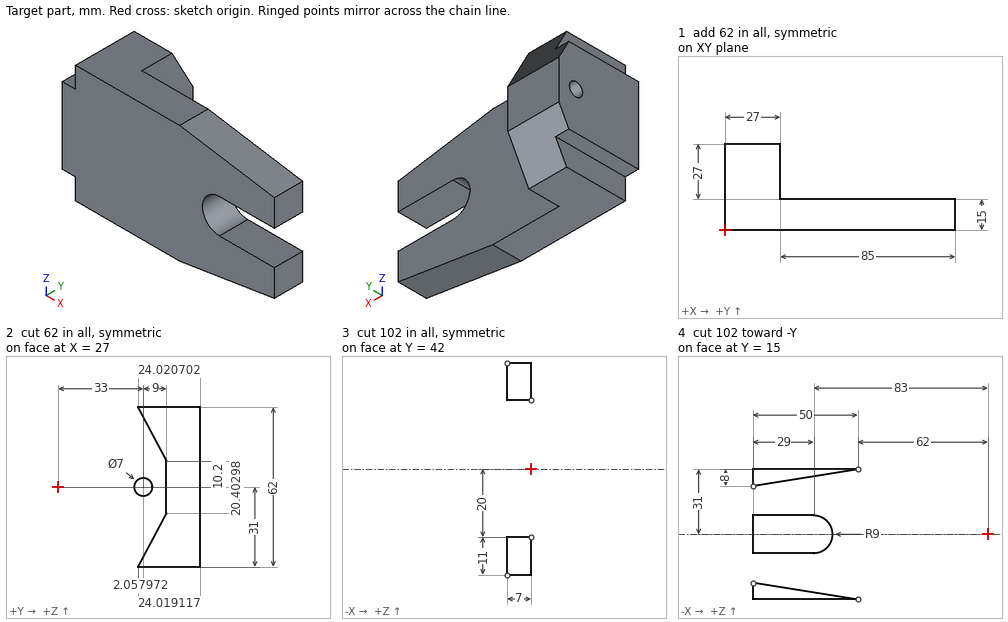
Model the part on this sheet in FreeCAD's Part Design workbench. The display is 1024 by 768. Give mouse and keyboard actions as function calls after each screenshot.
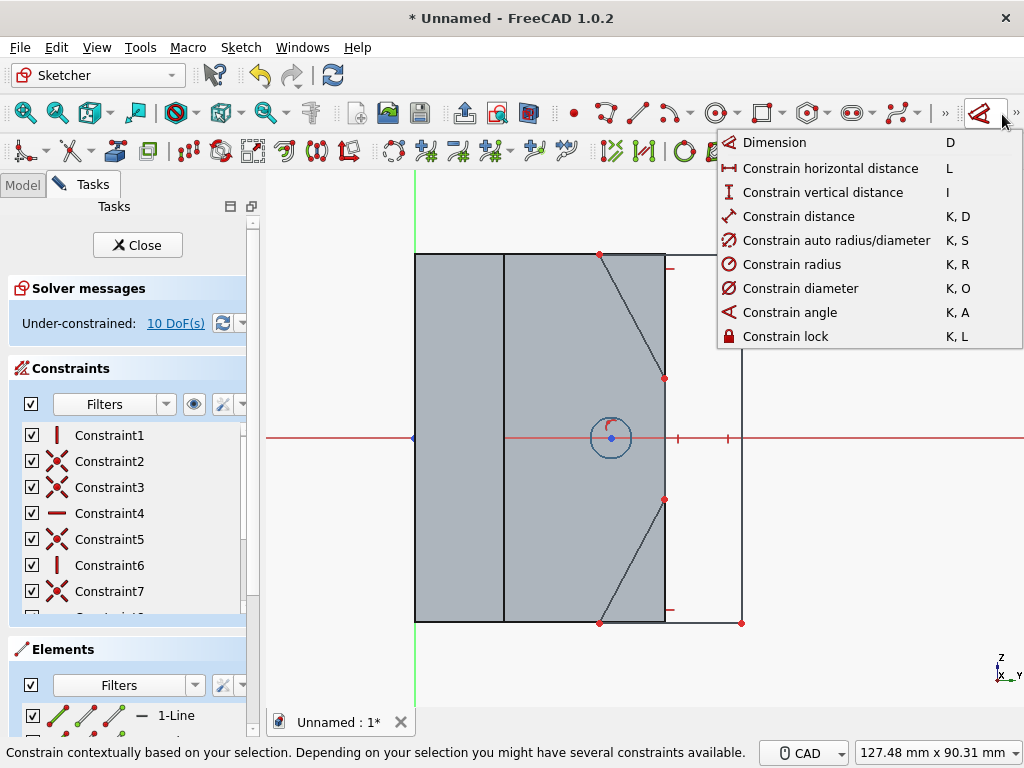
click(870, 288)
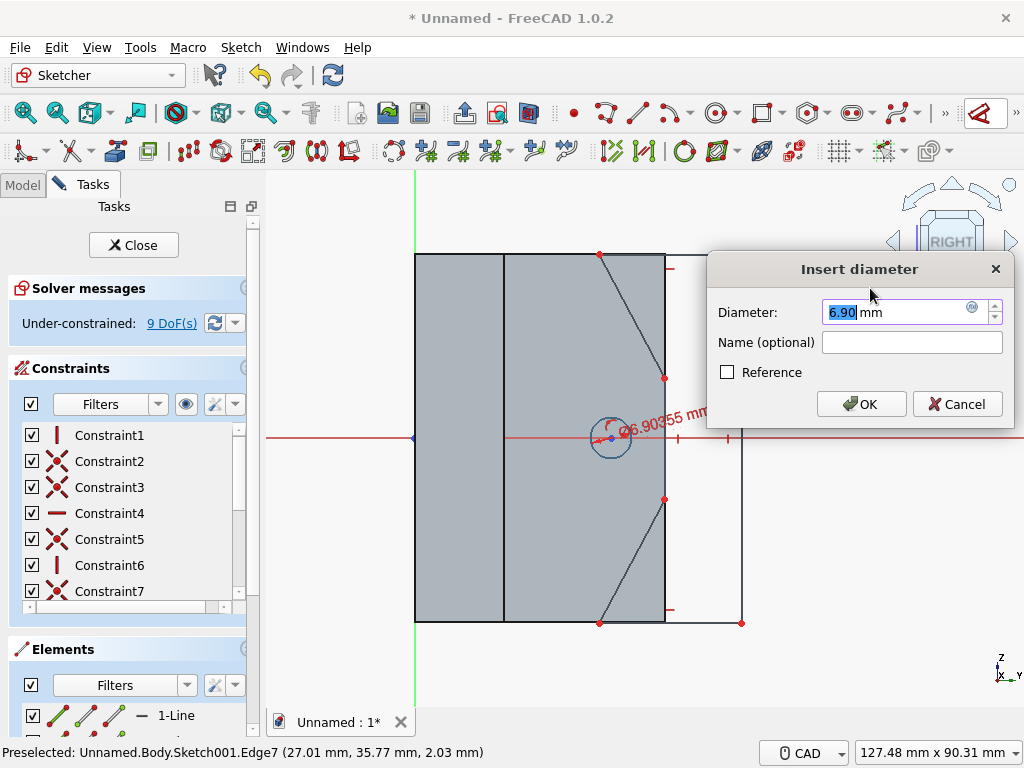
text(7)
key(Return)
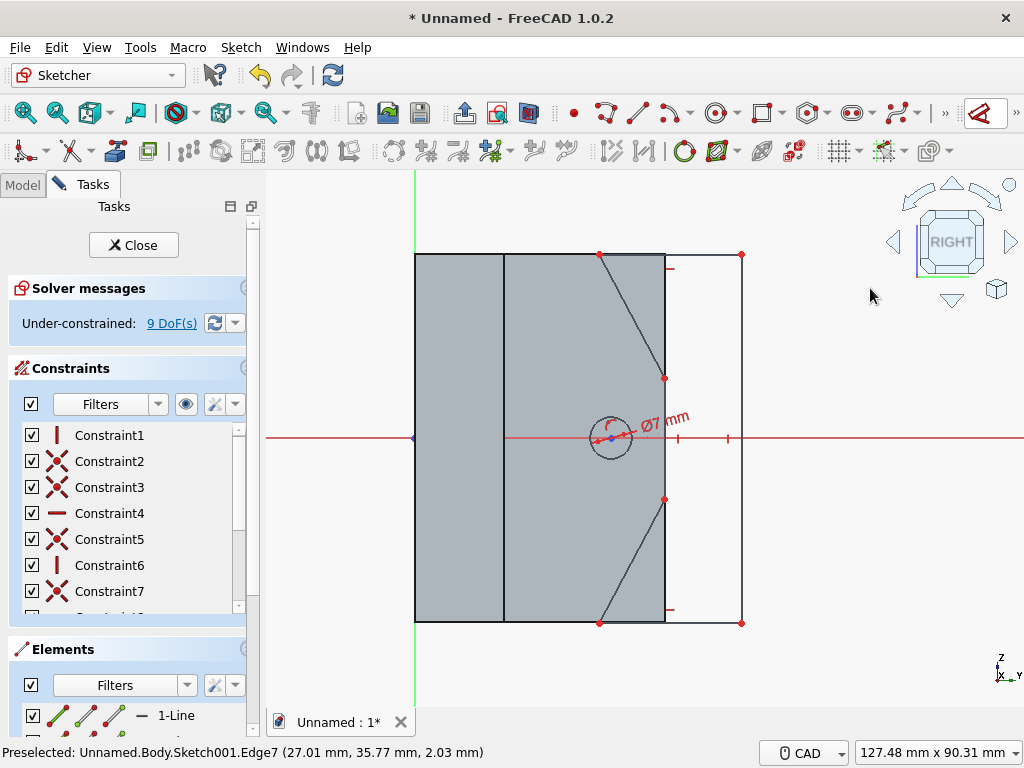
click(742, 513)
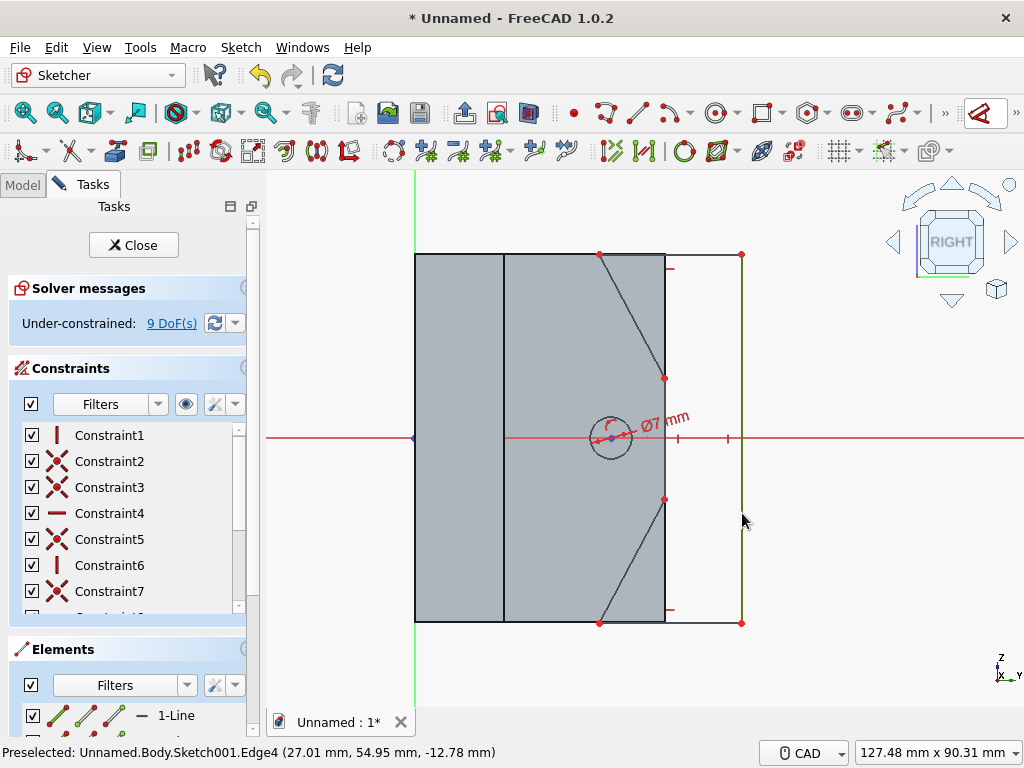
click(1002, 114)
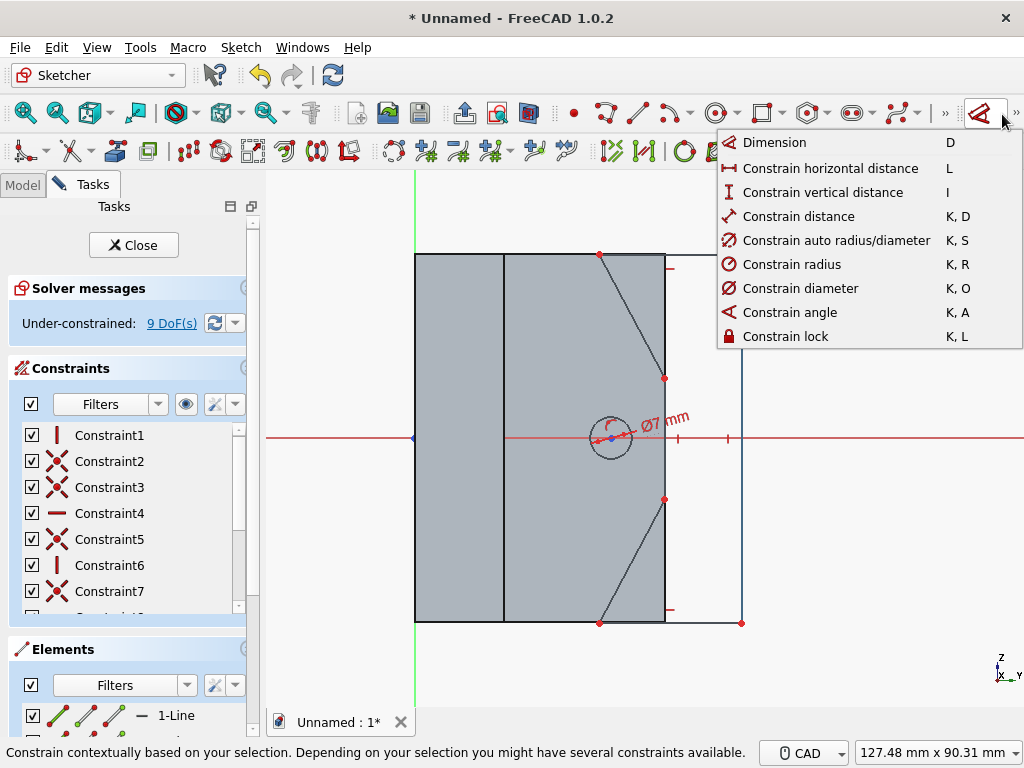
click(870, 192)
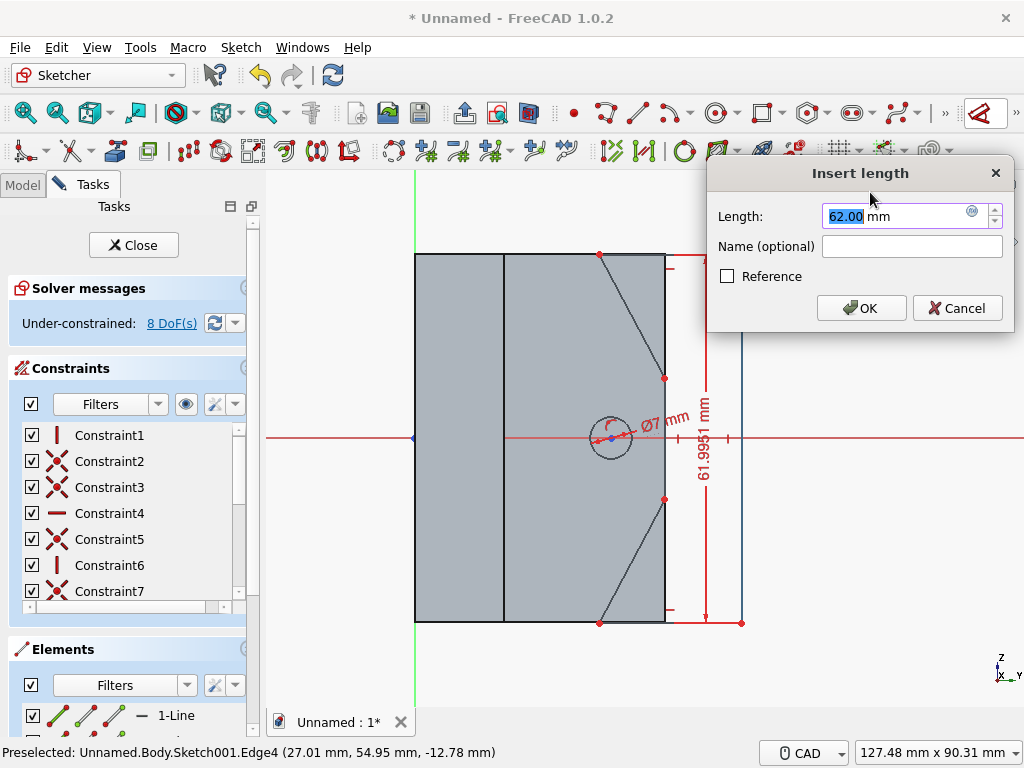
text(62)
key(Return)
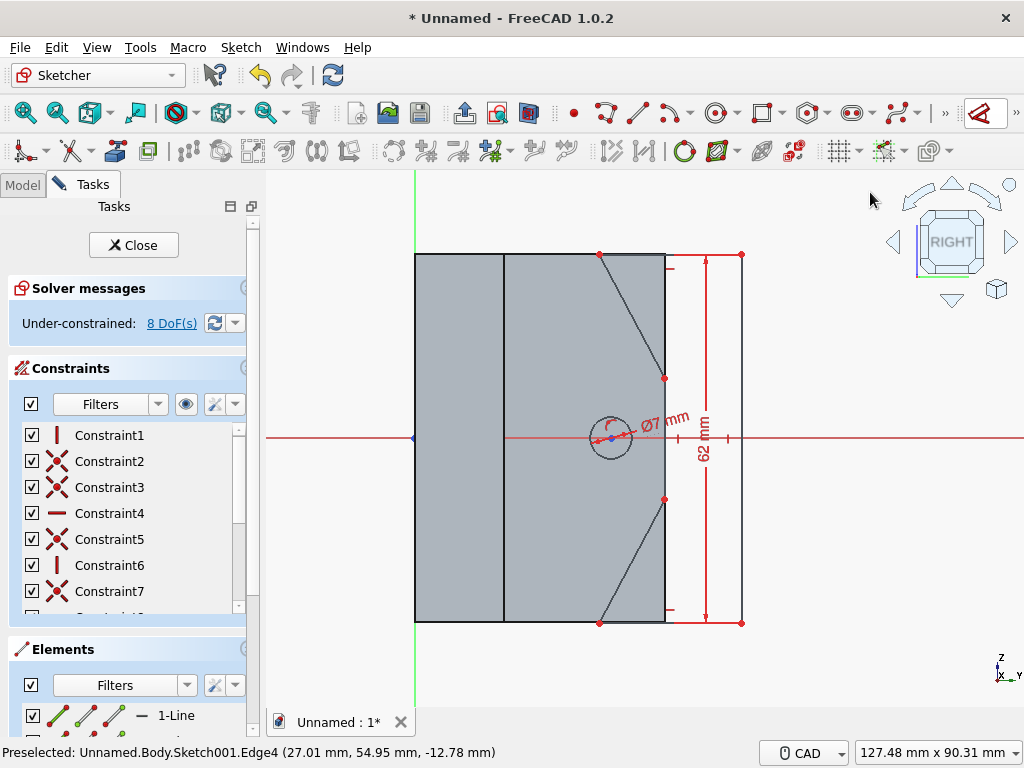
click(611, 438)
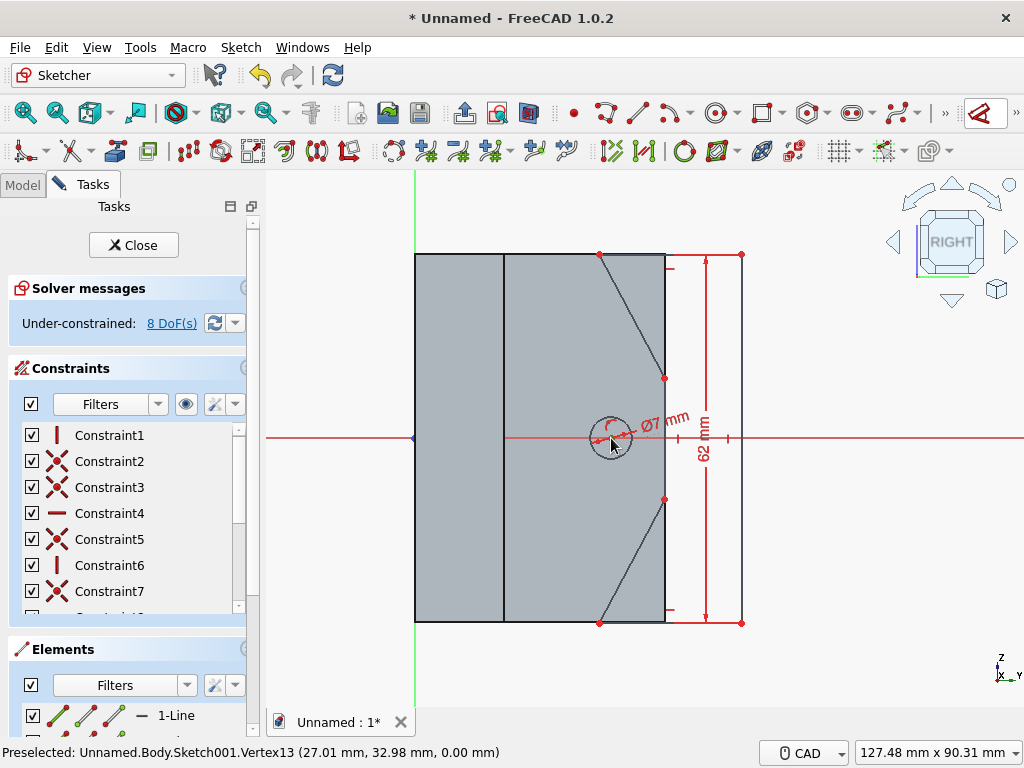
key(l)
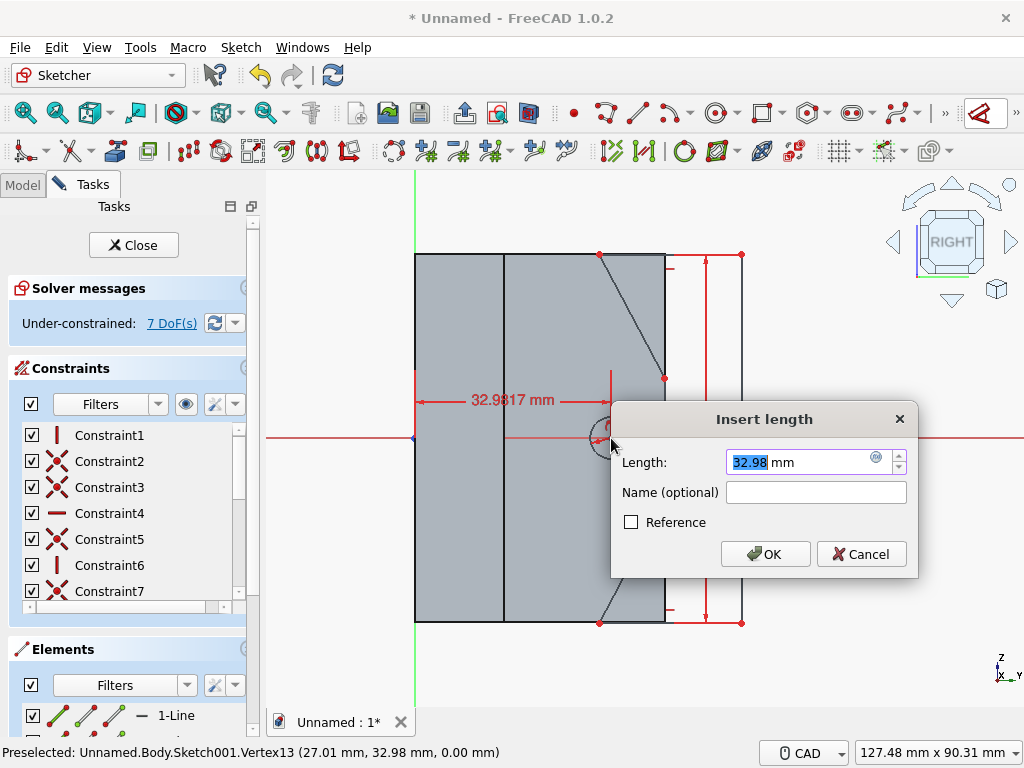
text(33)
key(Return)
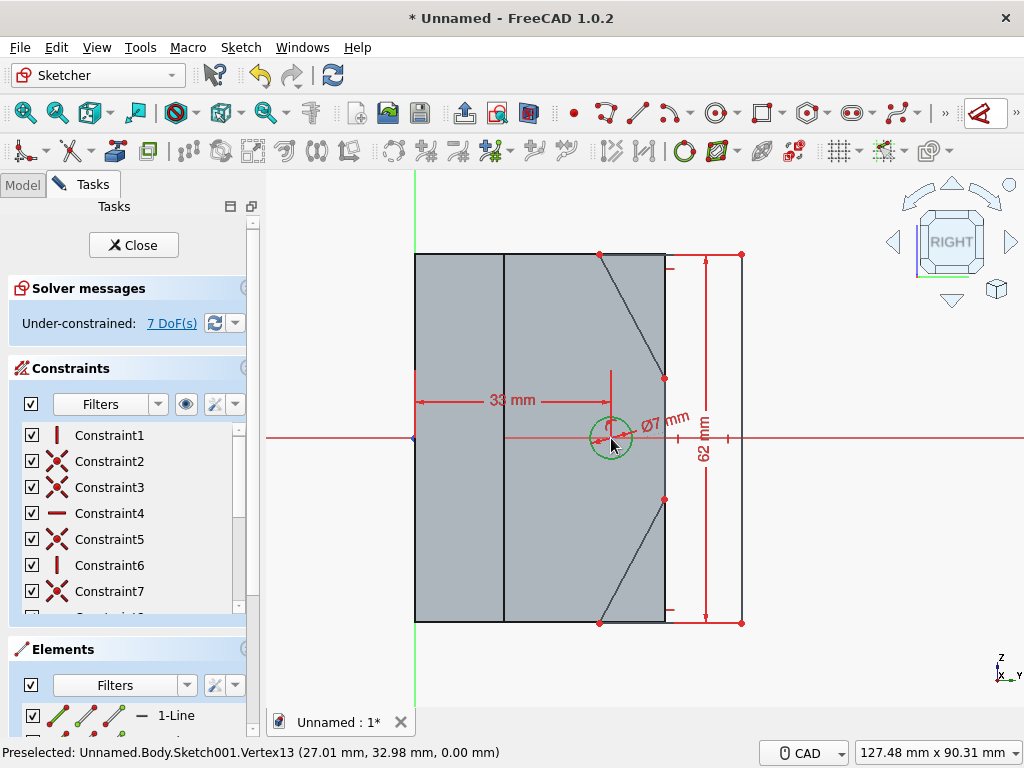
click(665, 378)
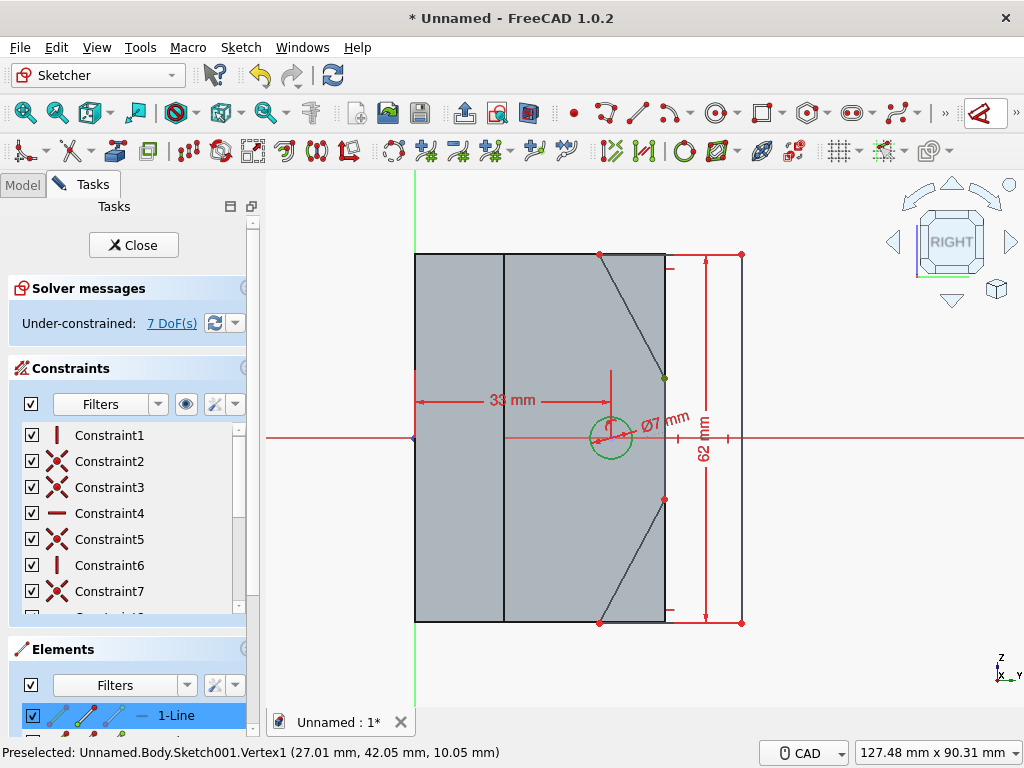
click(611, 438)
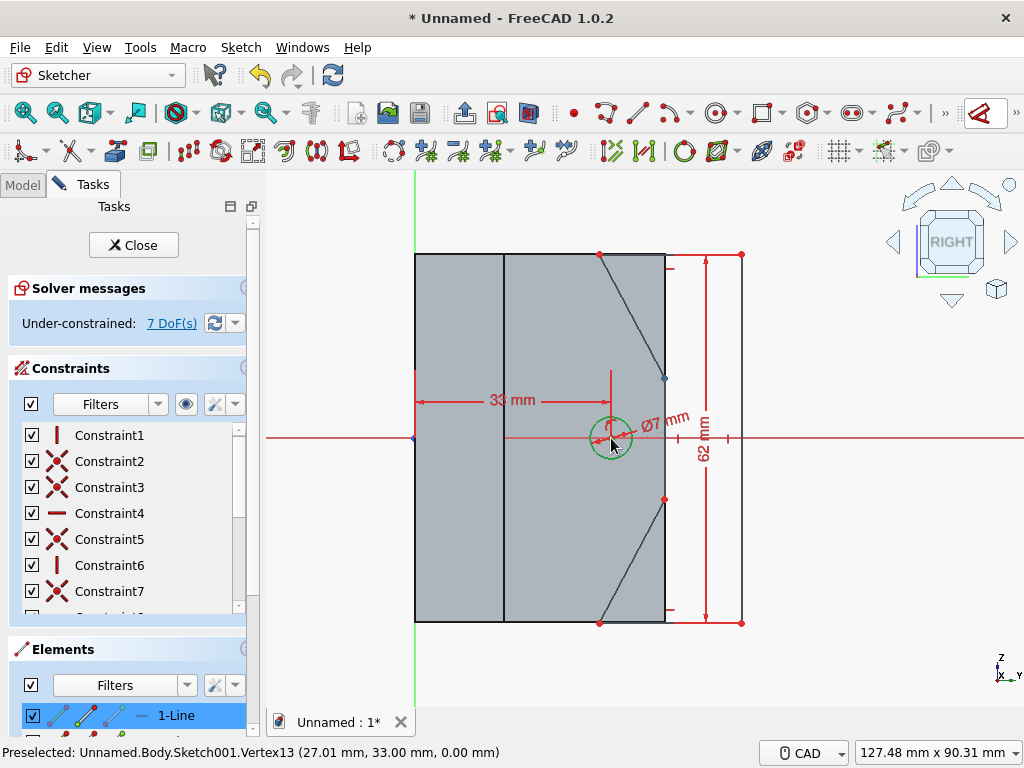
click(1002, 114)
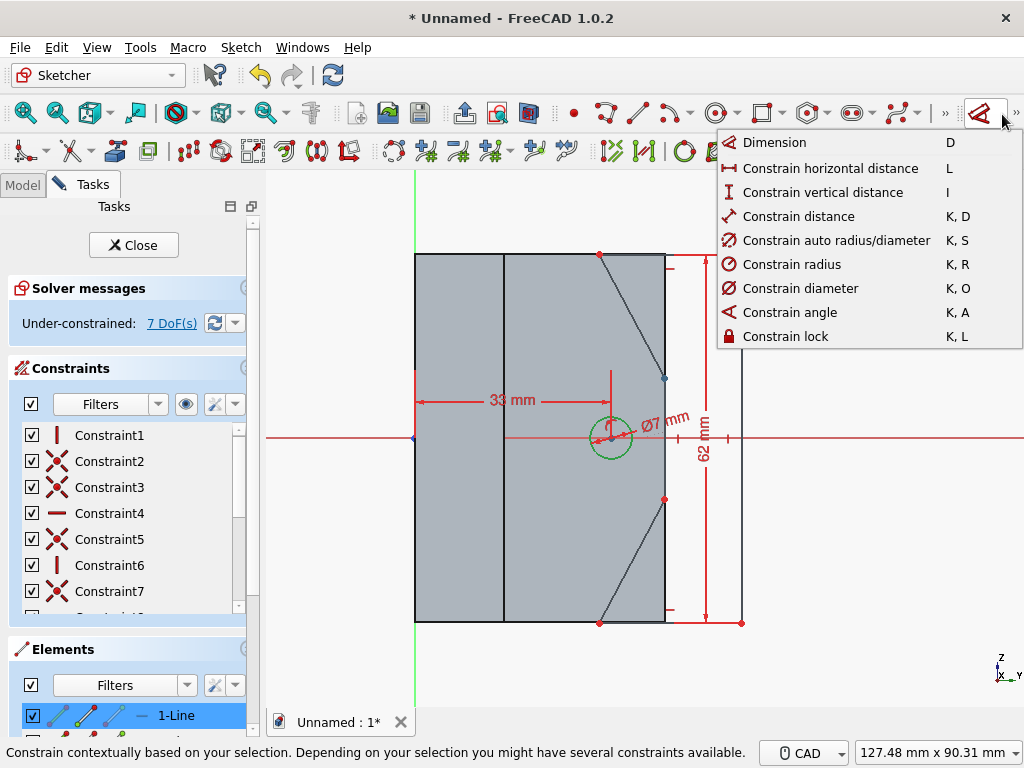
click(870, 168)